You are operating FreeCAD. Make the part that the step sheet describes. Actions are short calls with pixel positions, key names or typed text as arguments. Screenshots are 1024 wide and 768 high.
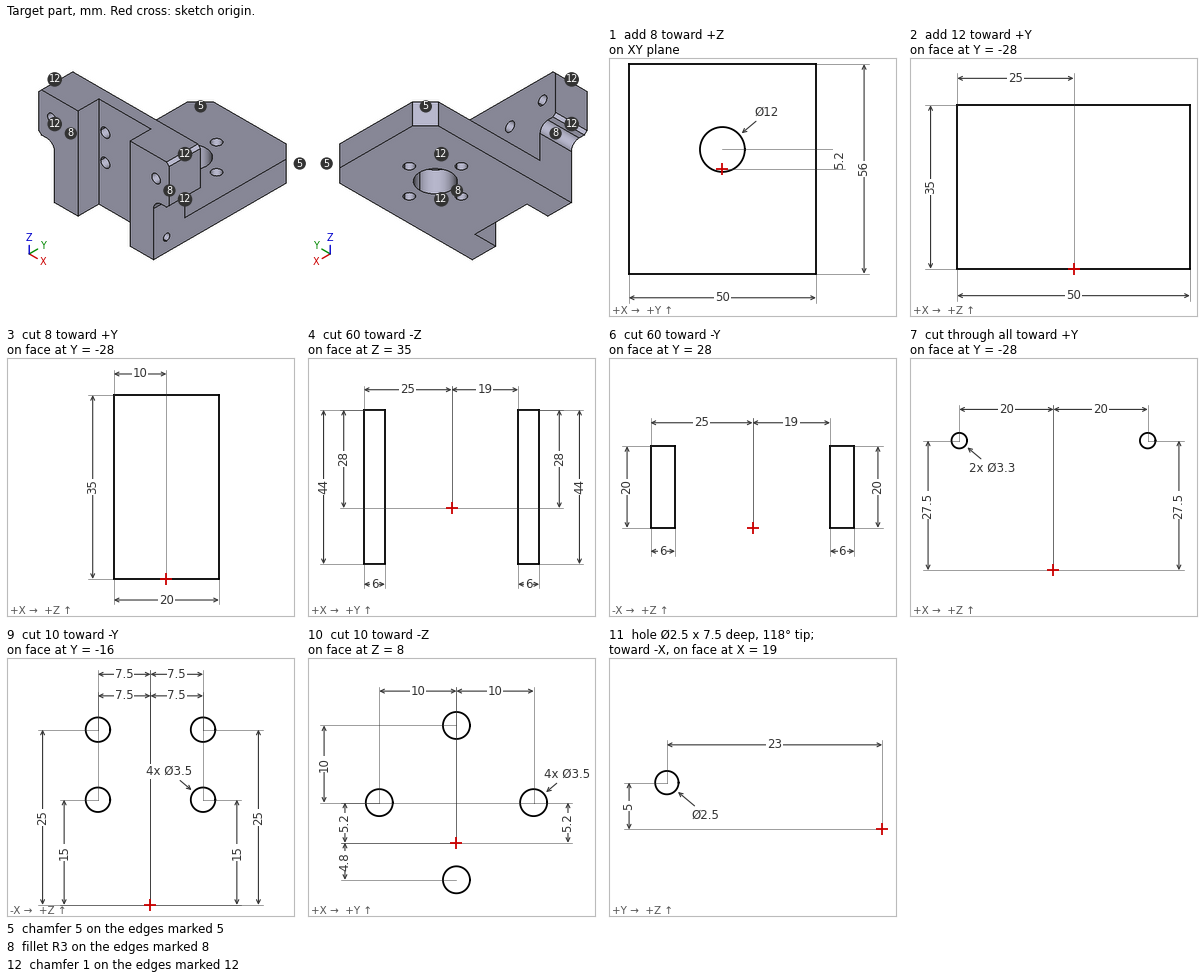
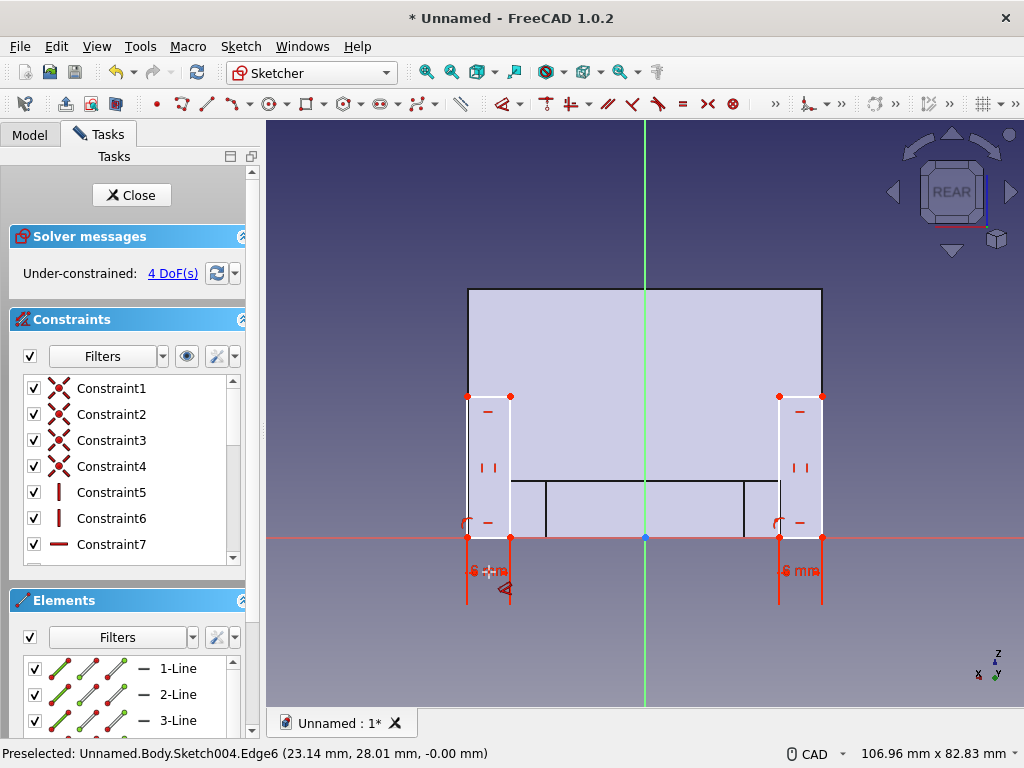
click(779, 439)
click(745, 467)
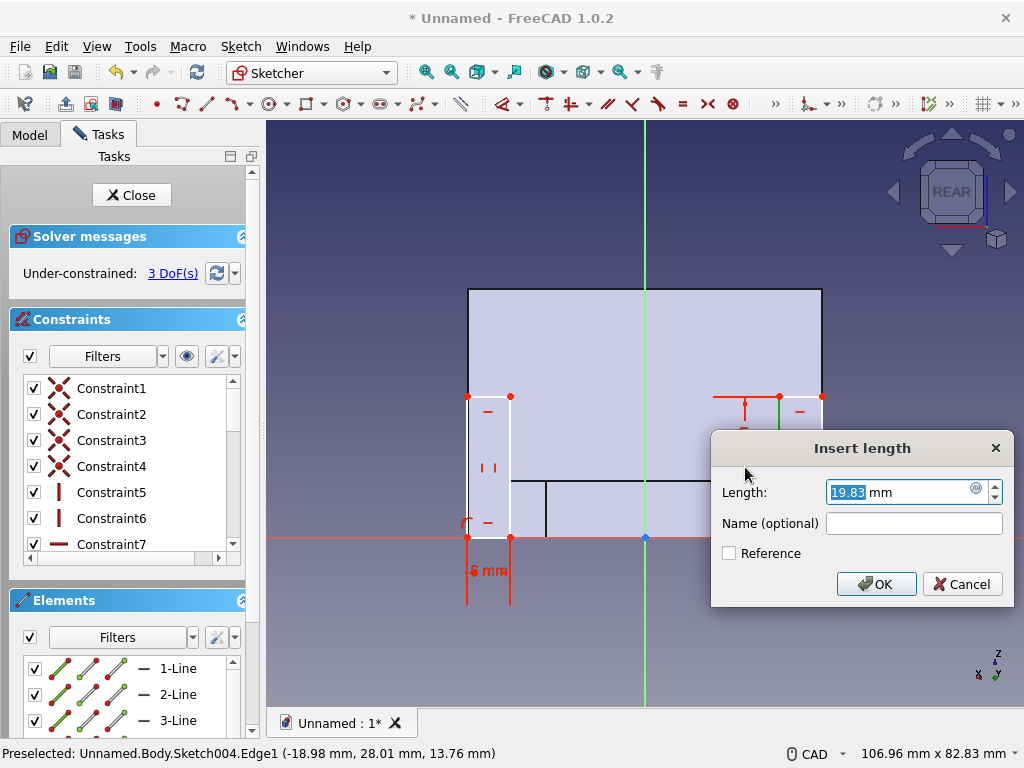
text(20)
key(Return)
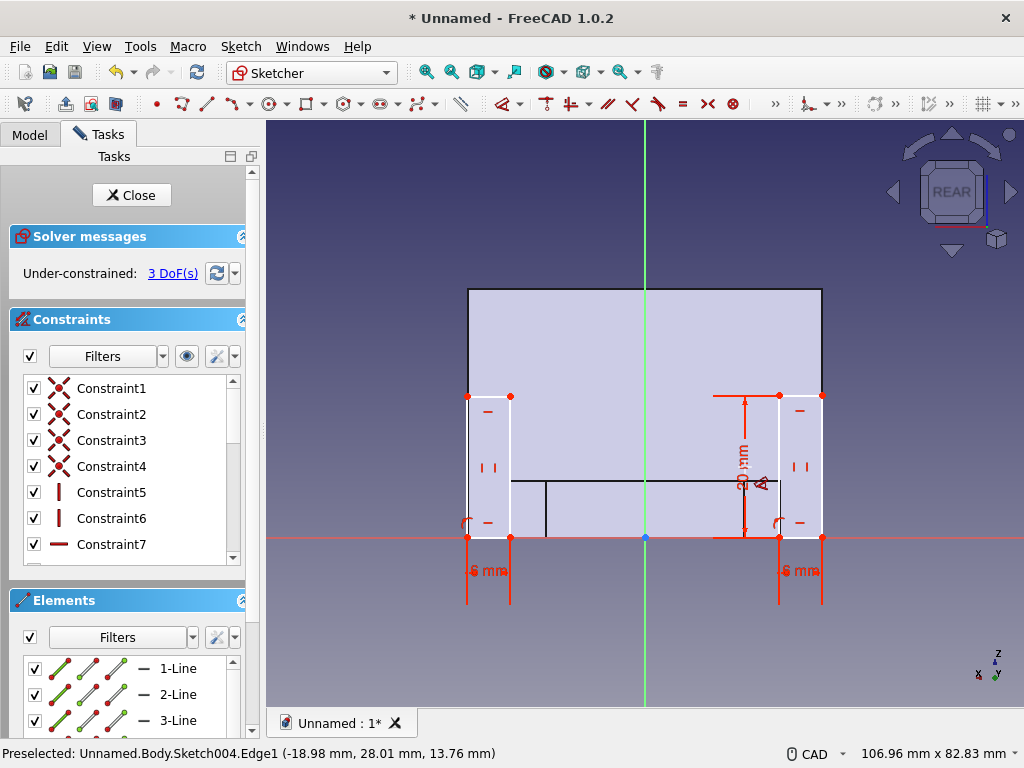
click(467, 439)
click(433, 467)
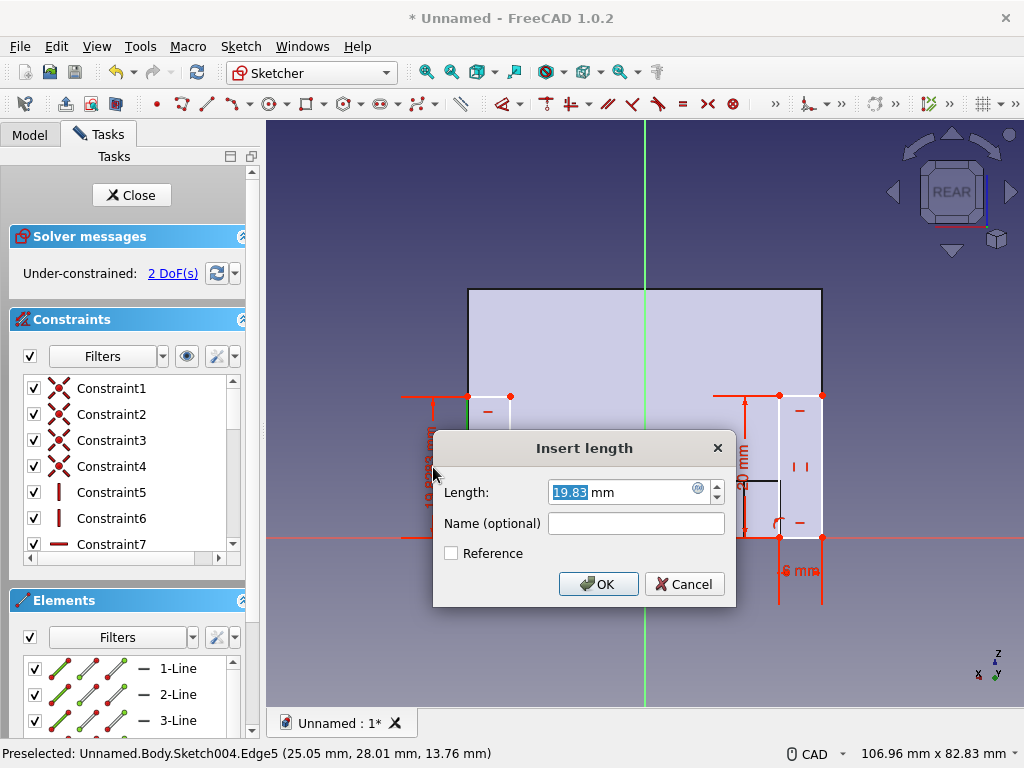
text(20)
key(Return)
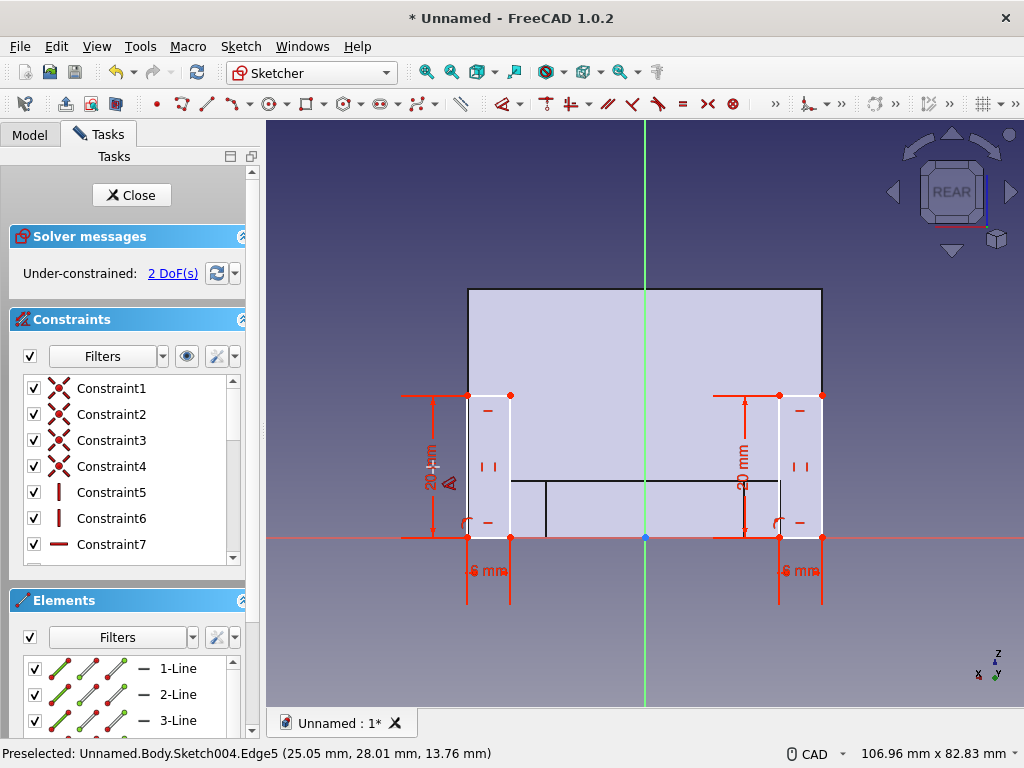
click(779, 396)
click(712, 572)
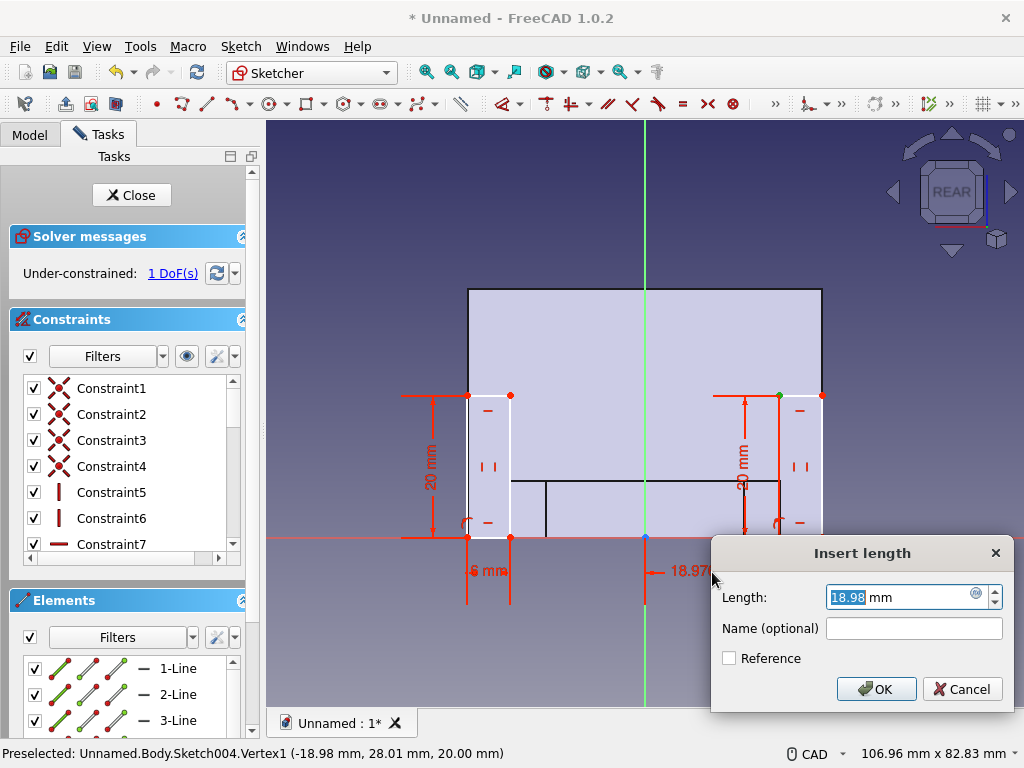
text(19)
key(Return)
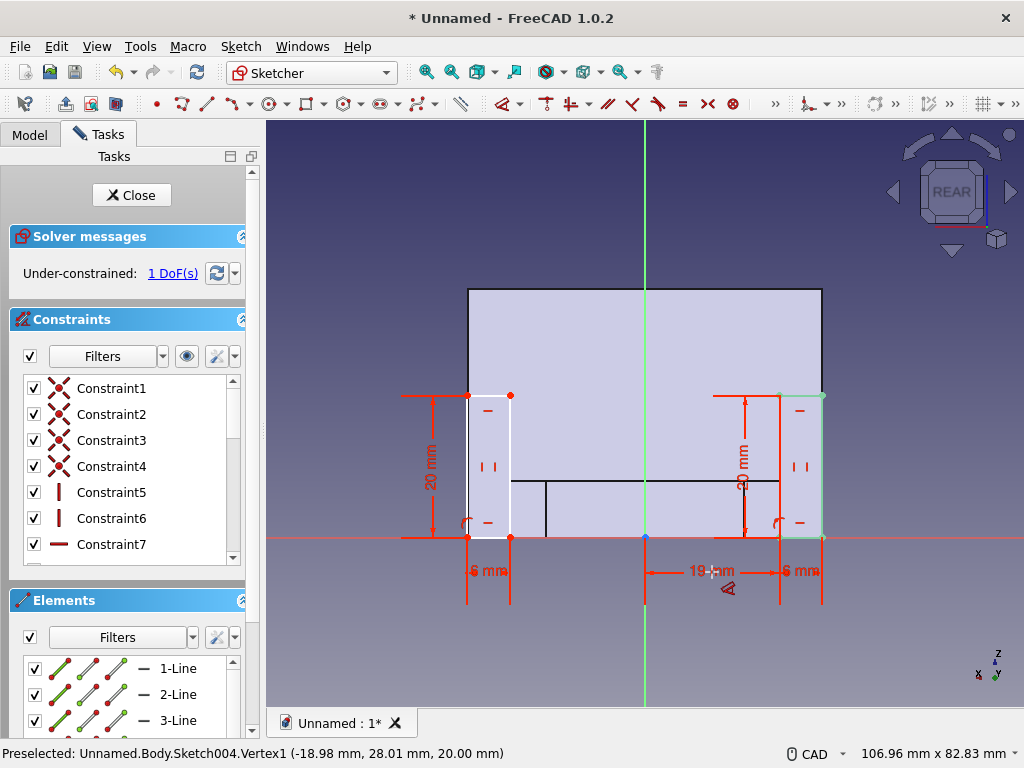
click(467, 396)
click(597, 572)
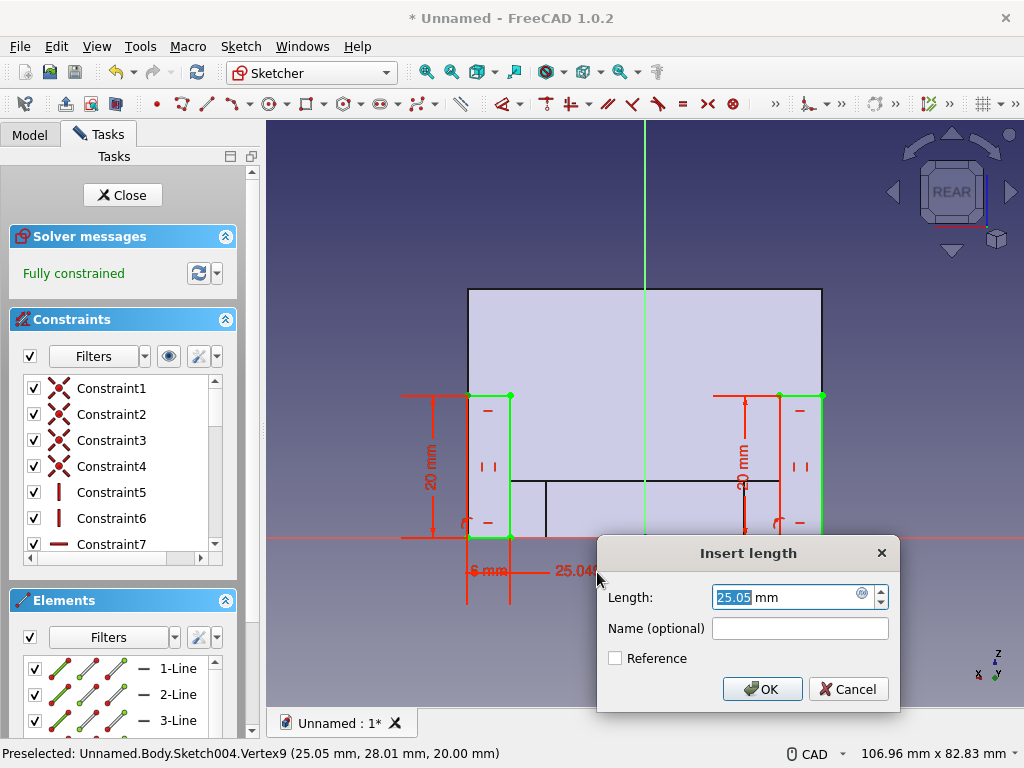
text(25)
key(Return)
key(Escape)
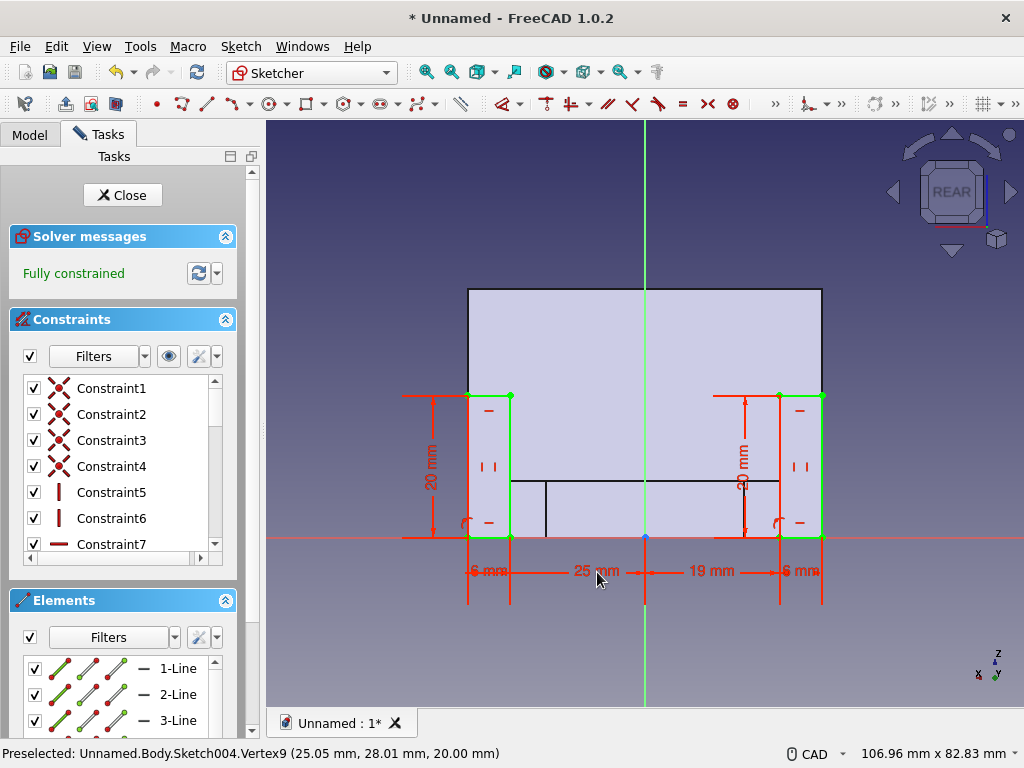
click(123, 195)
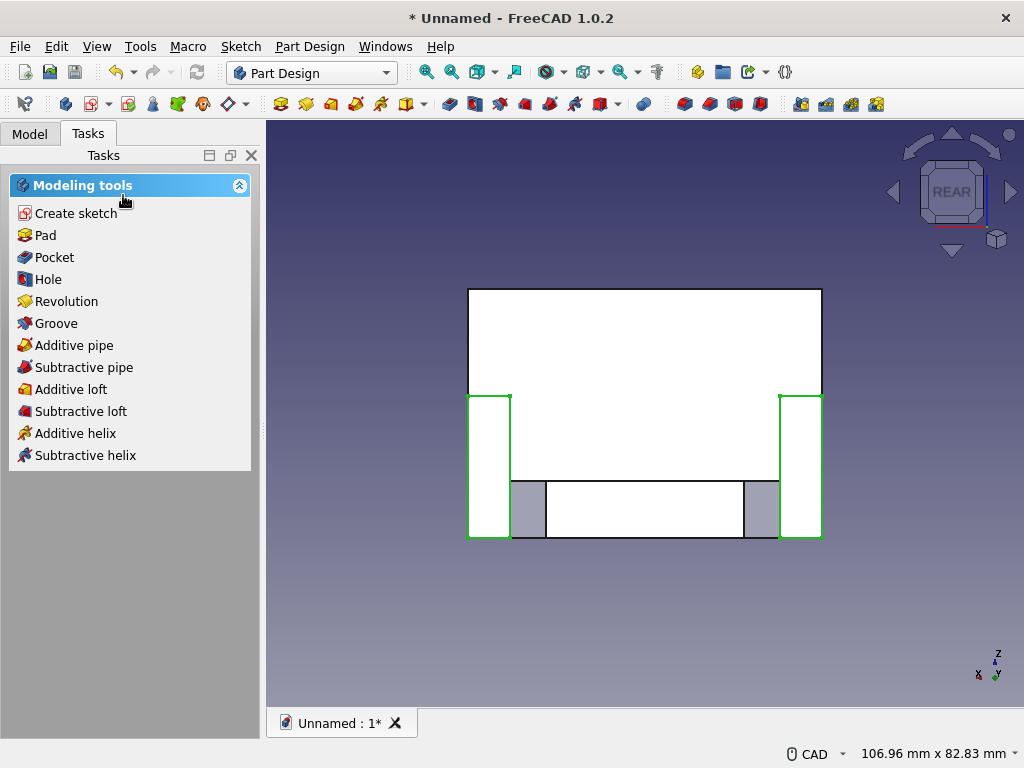
click(450, 104)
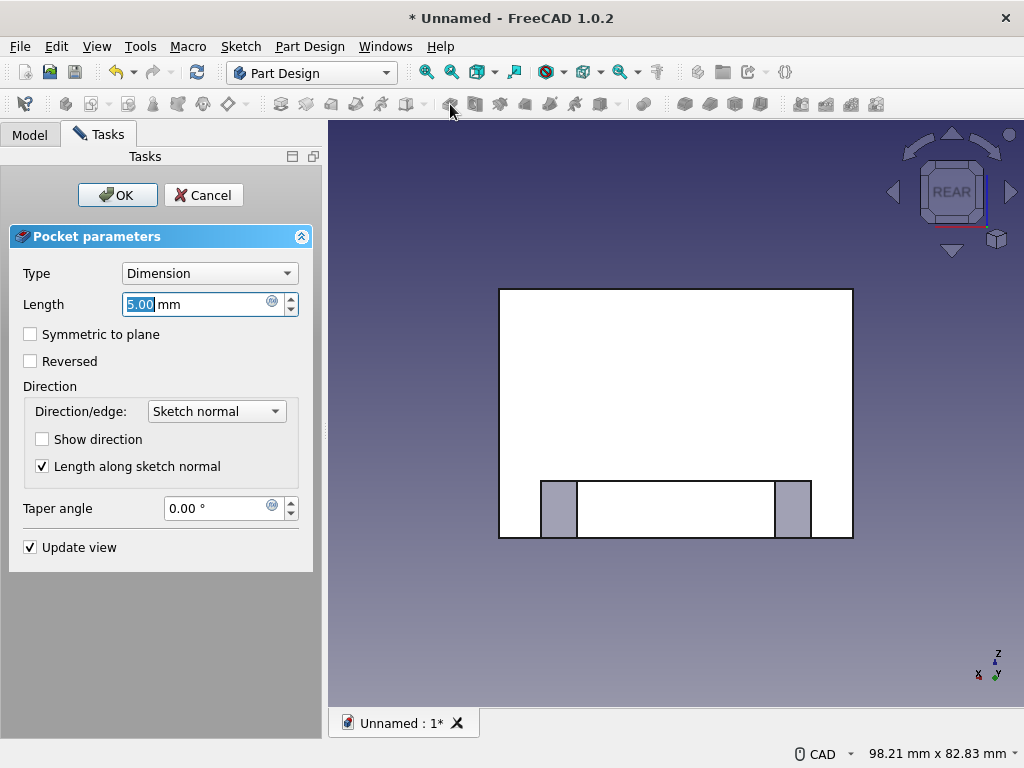
text(60)
key(Tab)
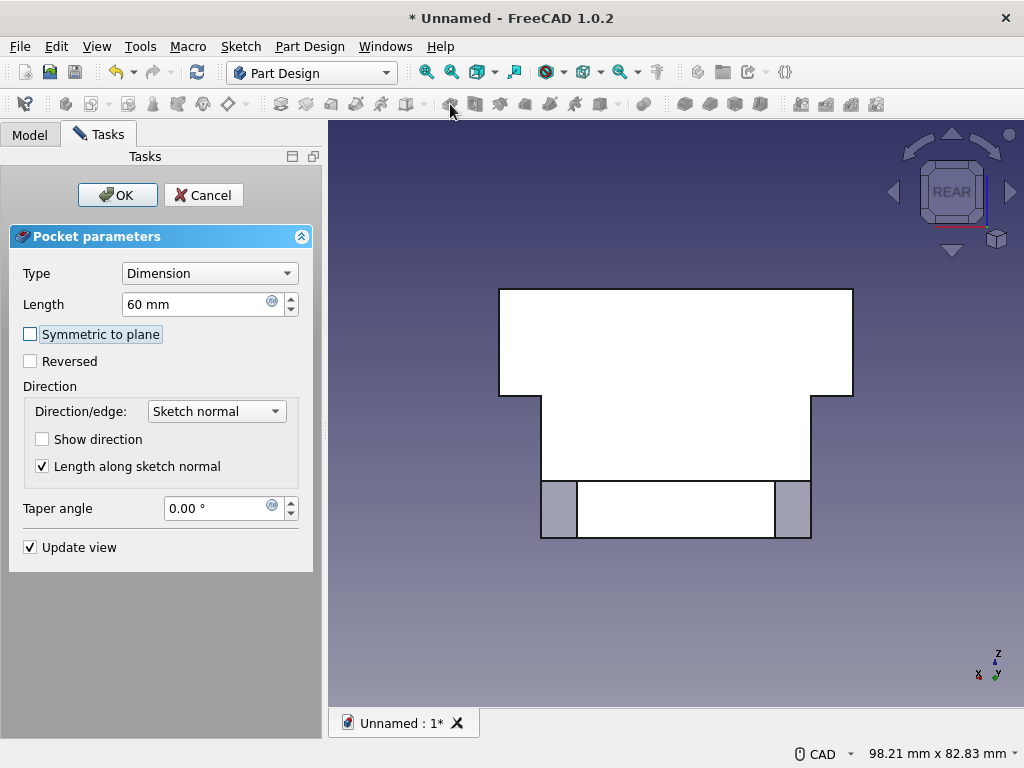
click(118, 195)